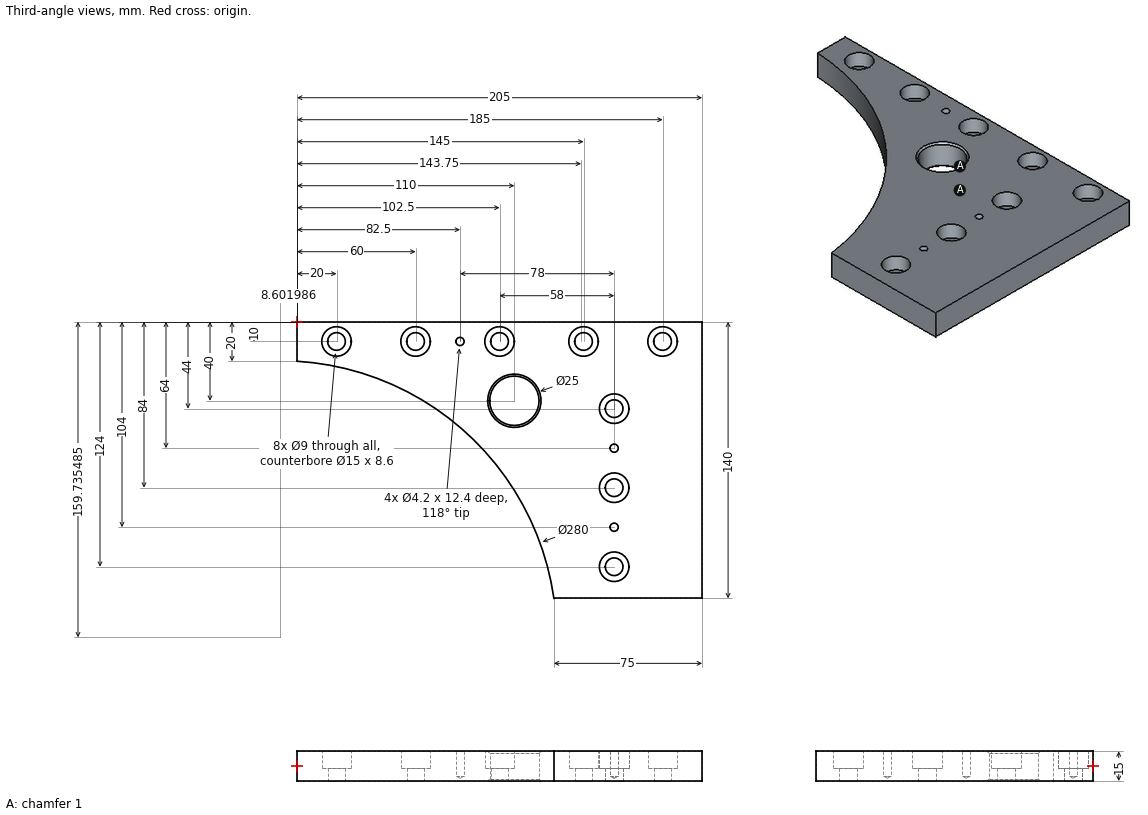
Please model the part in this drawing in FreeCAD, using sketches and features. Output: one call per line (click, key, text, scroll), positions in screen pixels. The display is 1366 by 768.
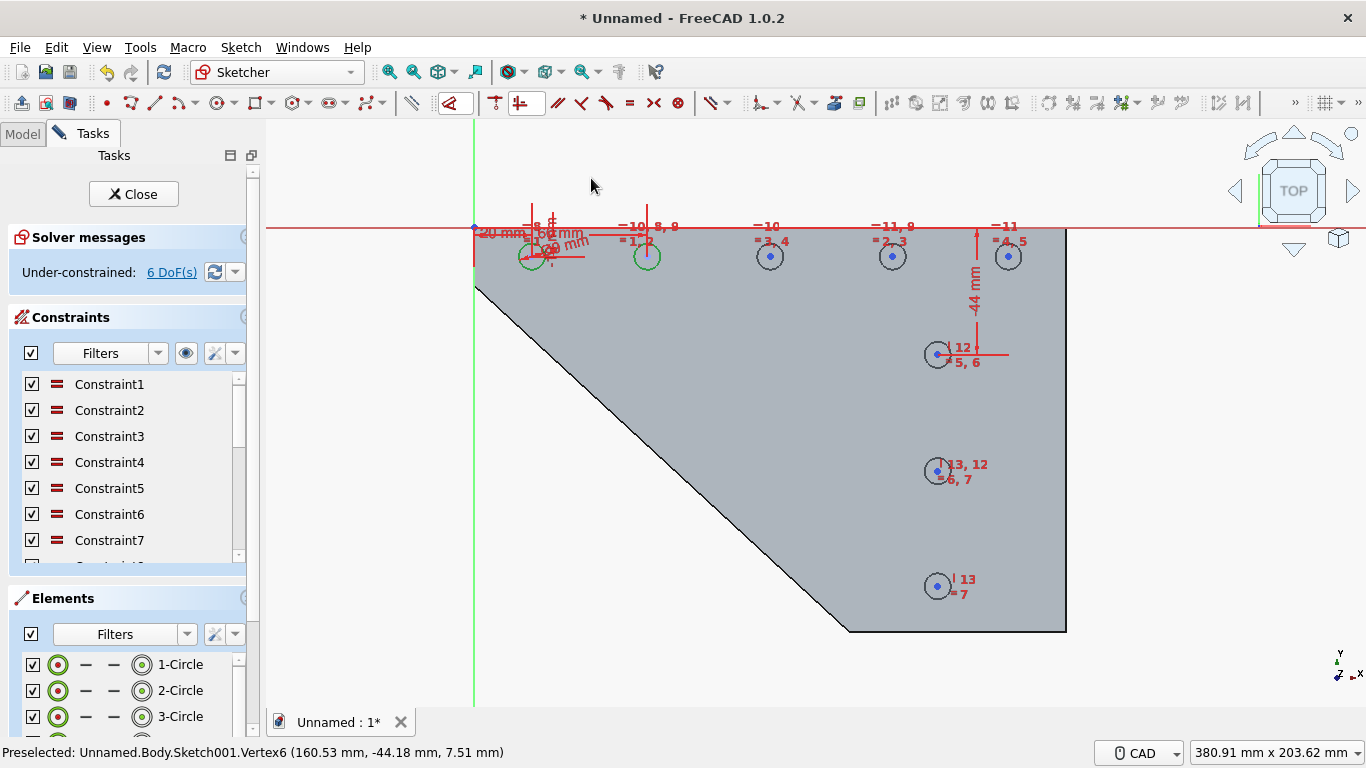
click(938, 471)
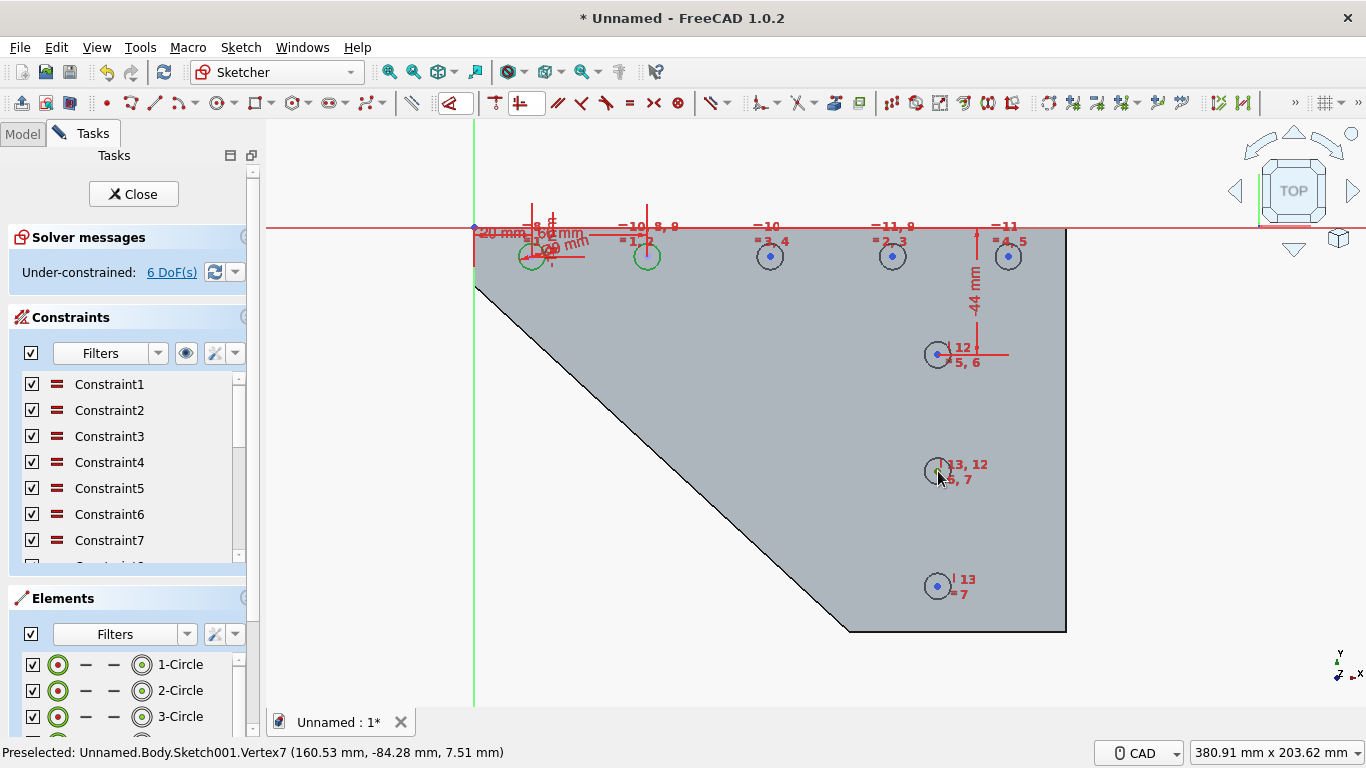
key(i)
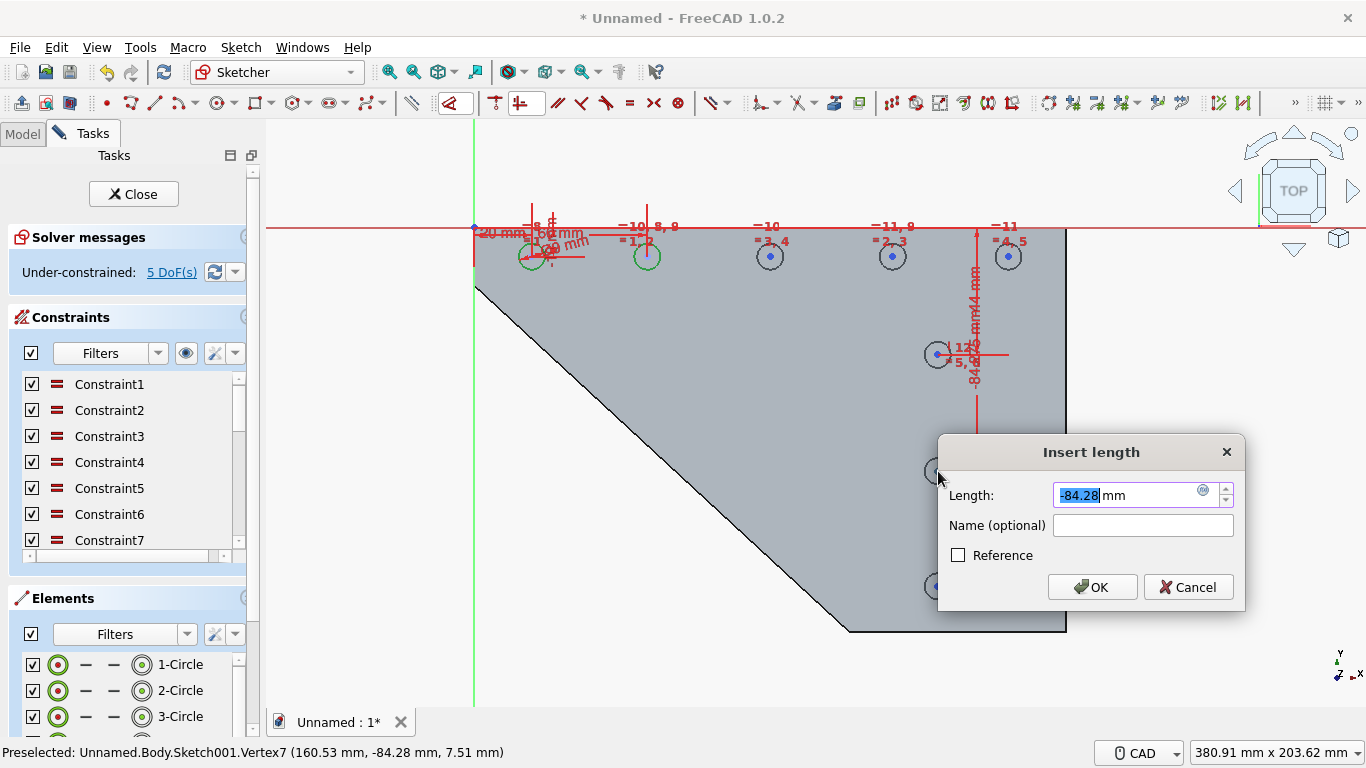
text(-84)
key(Return)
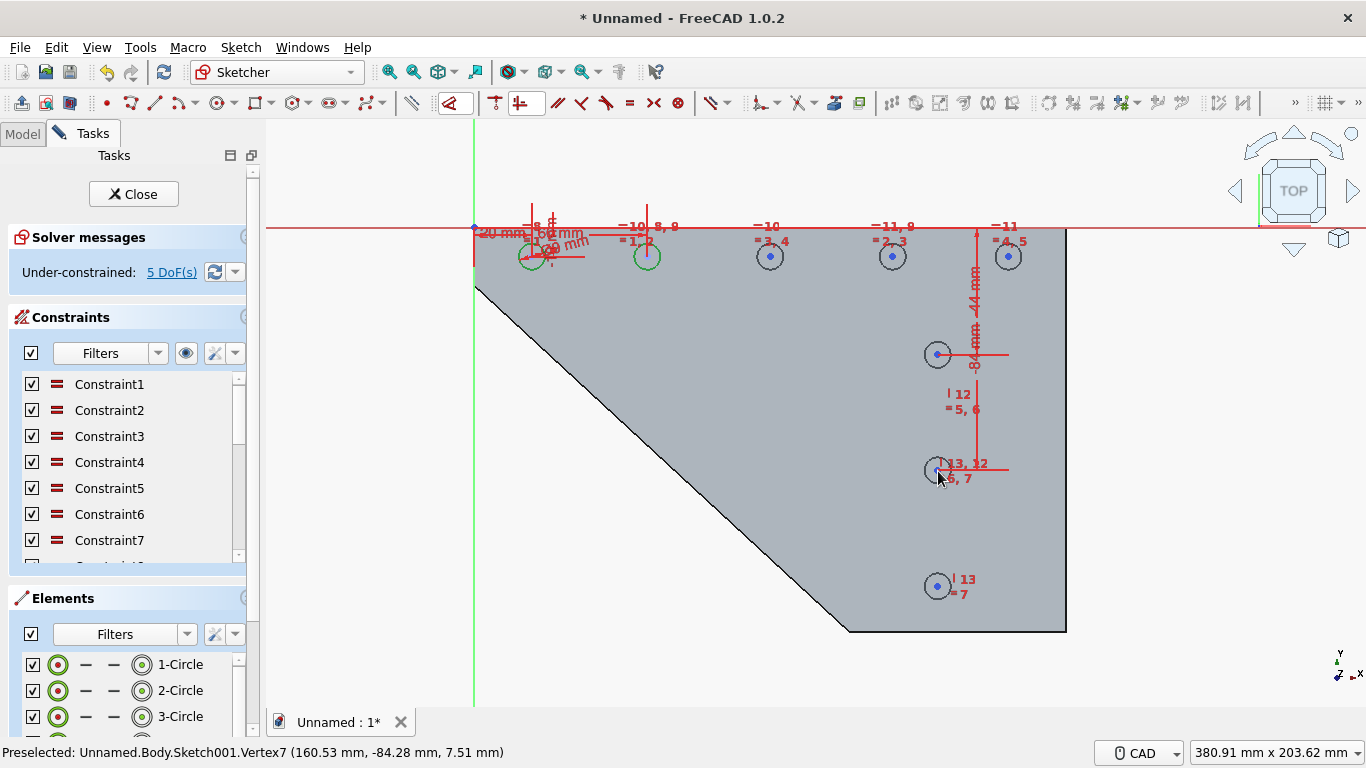
click(893, 257)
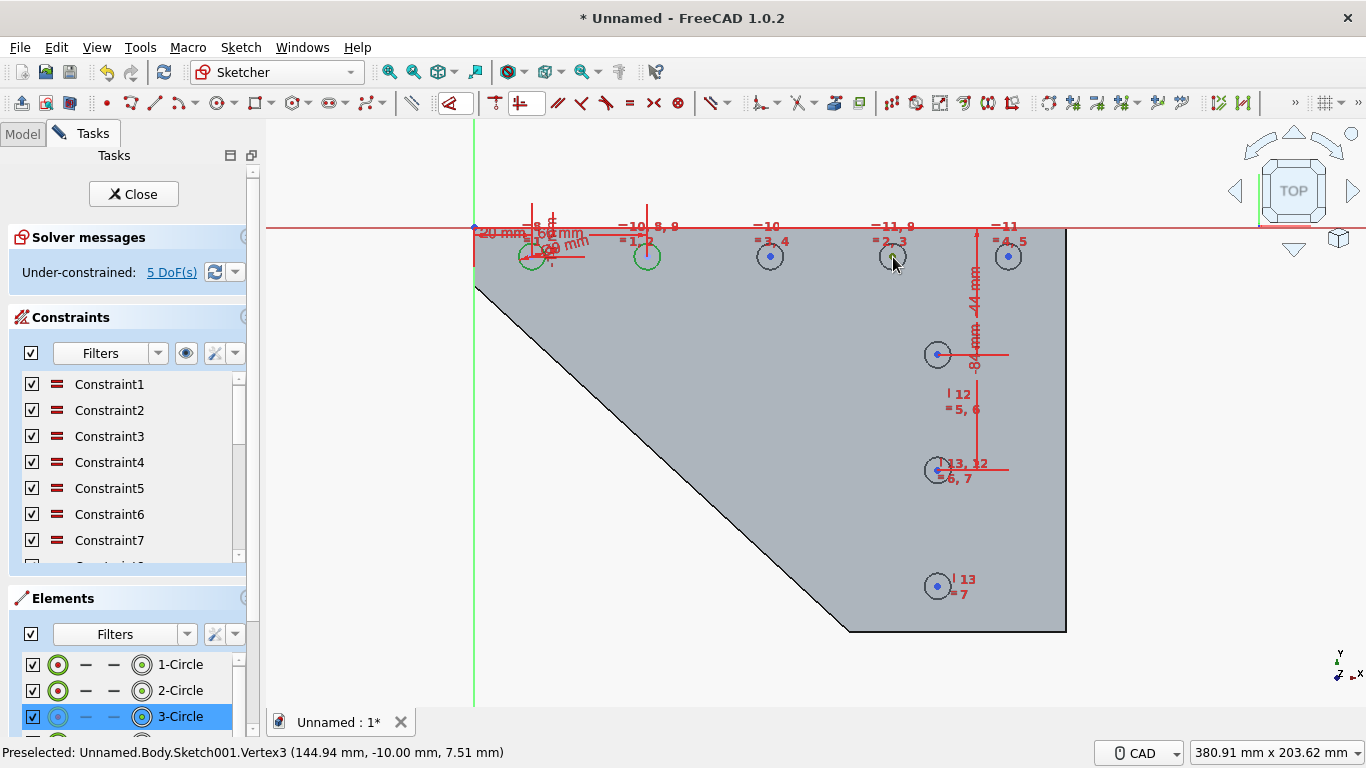
click(468, 104)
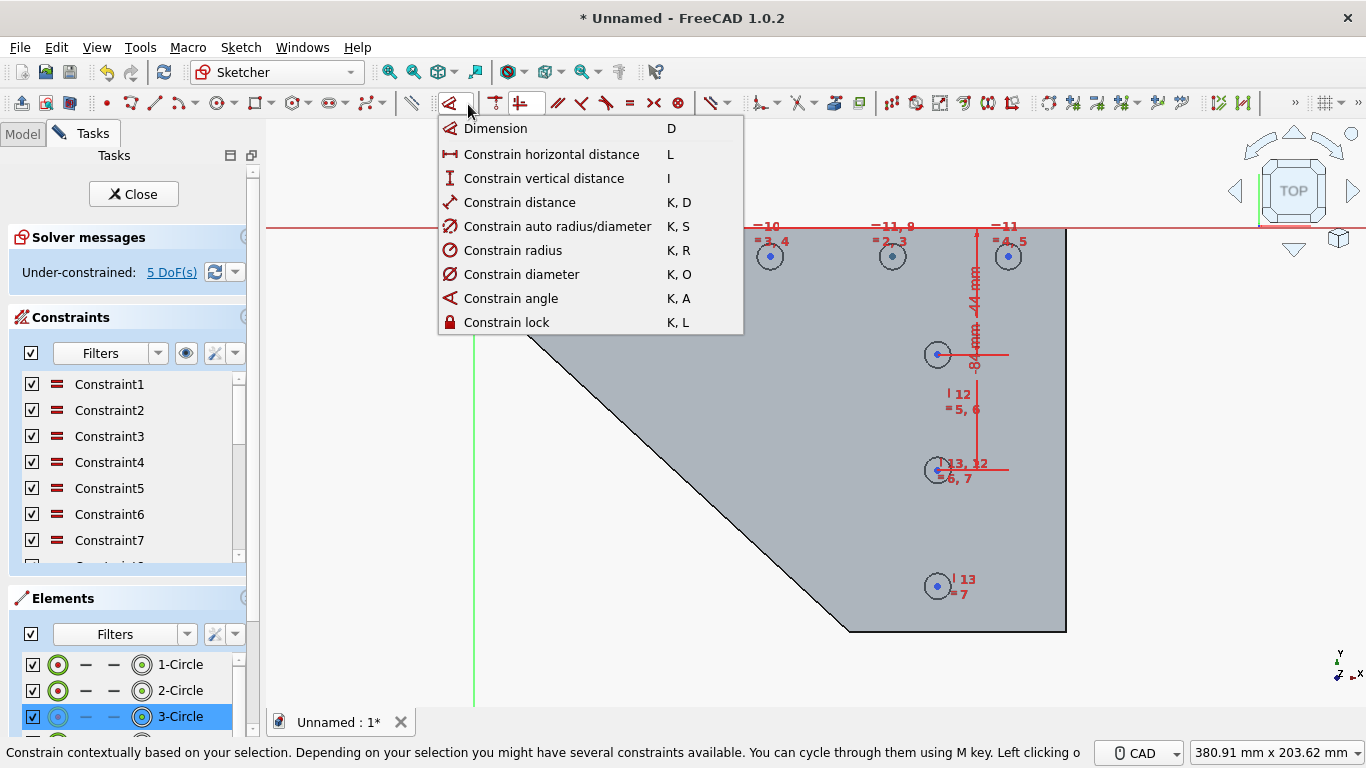
click(591, 154)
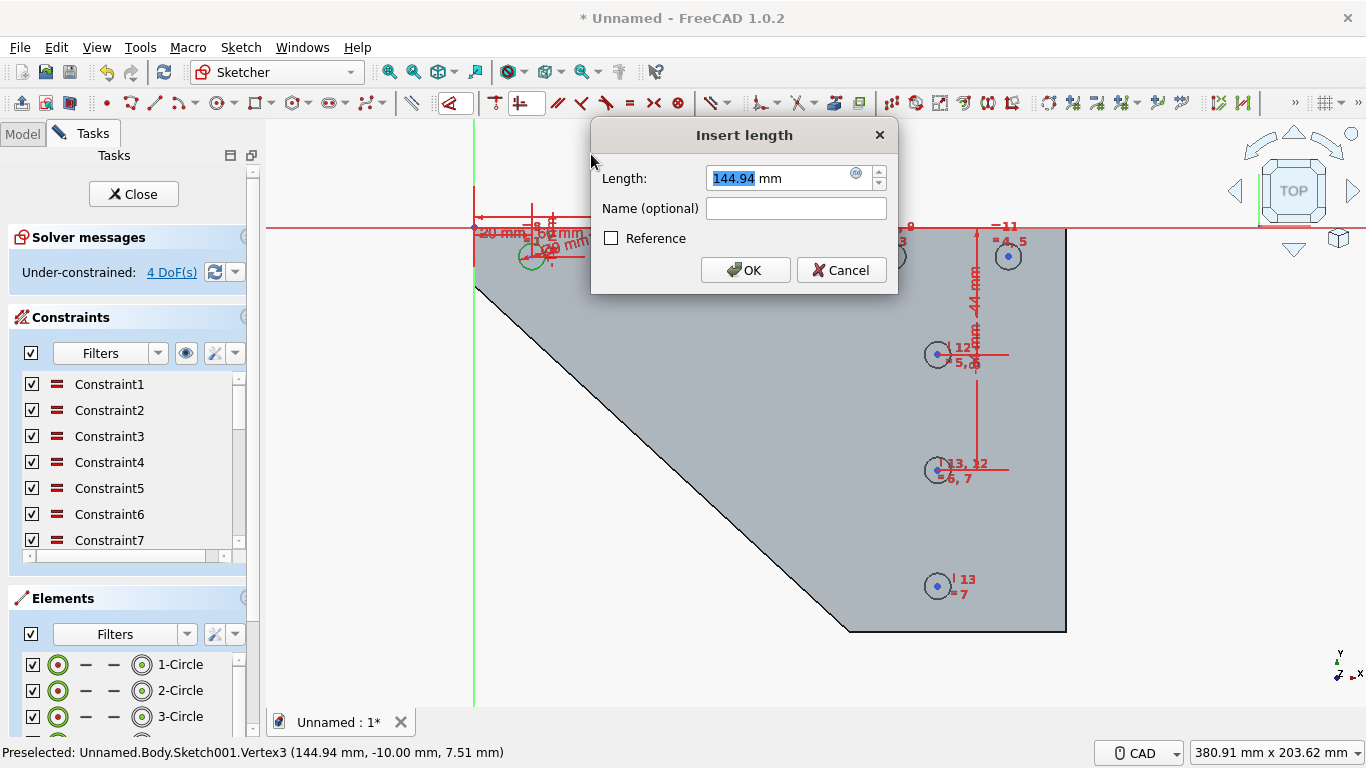
text(145)
key(Return)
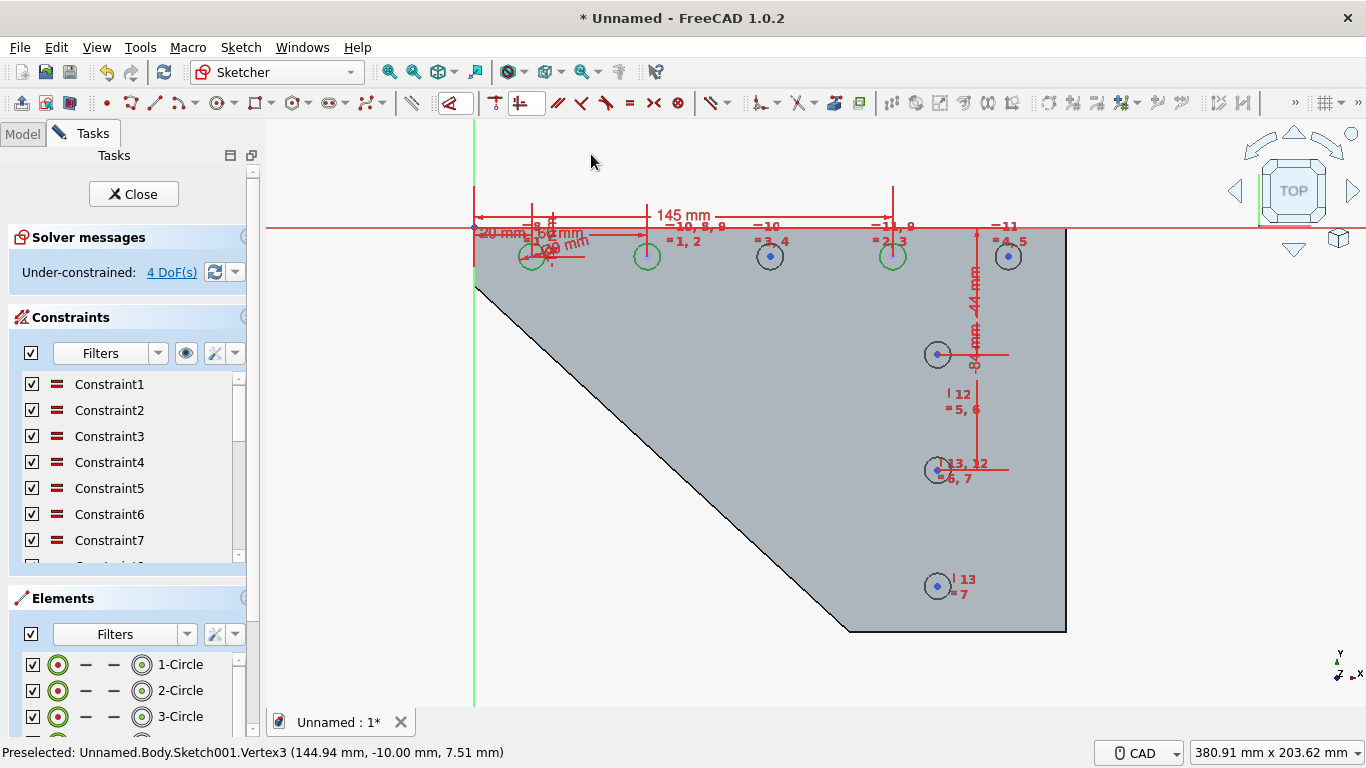
click(1009, 257)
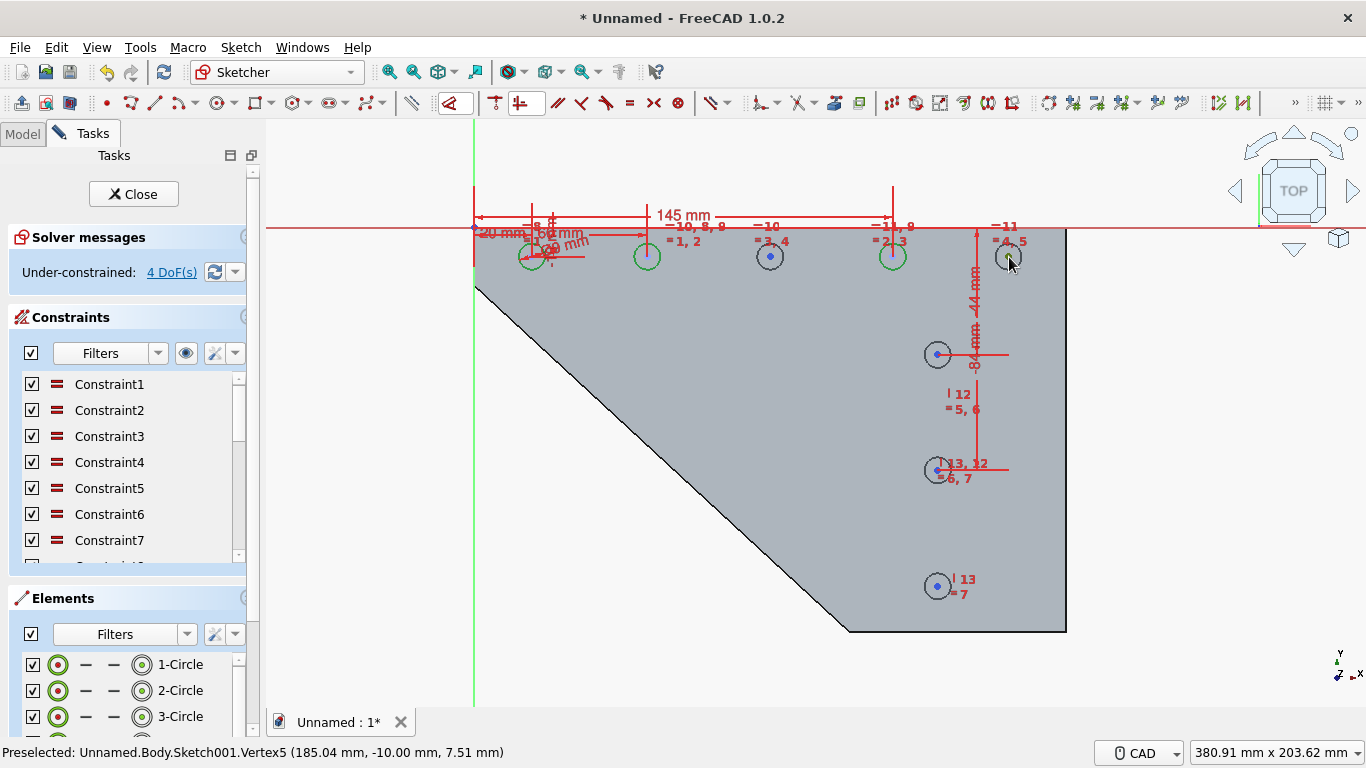
click(468, 104)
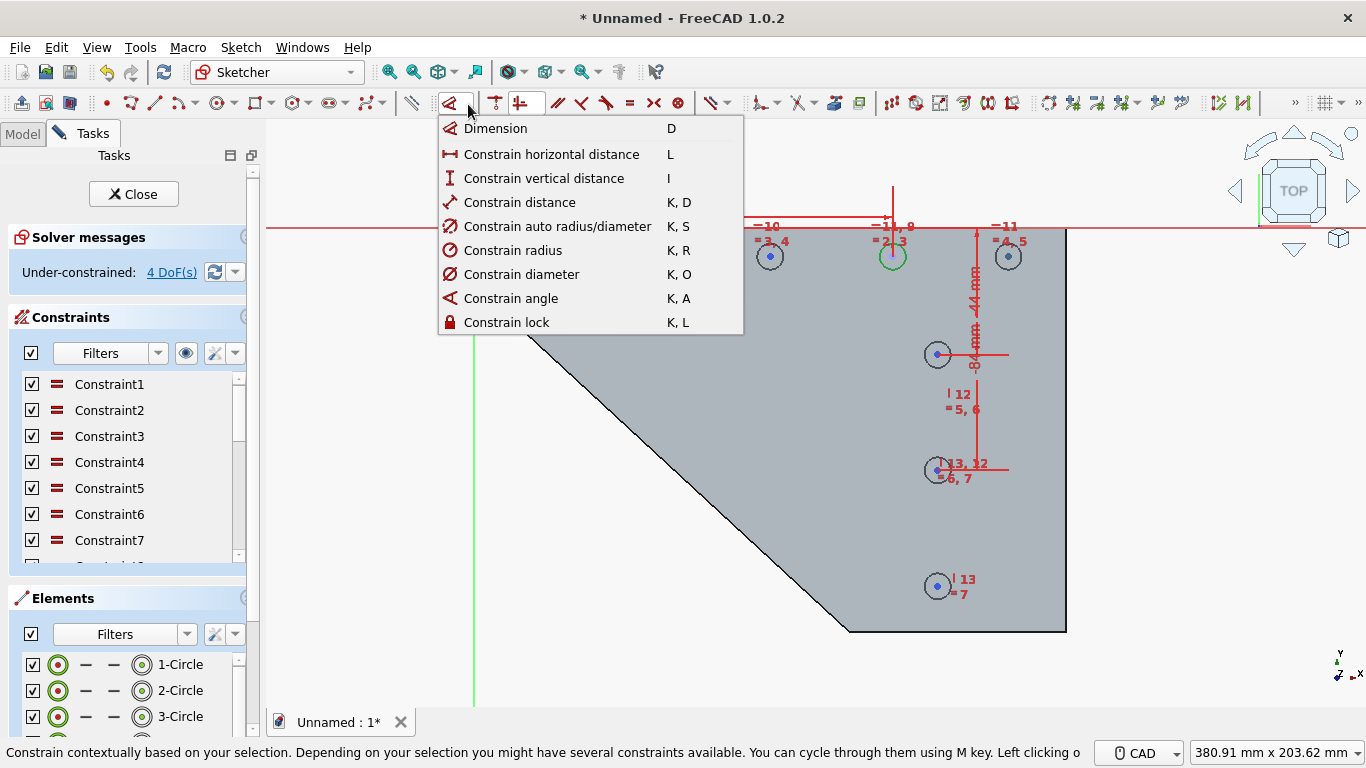
click(591, 154)